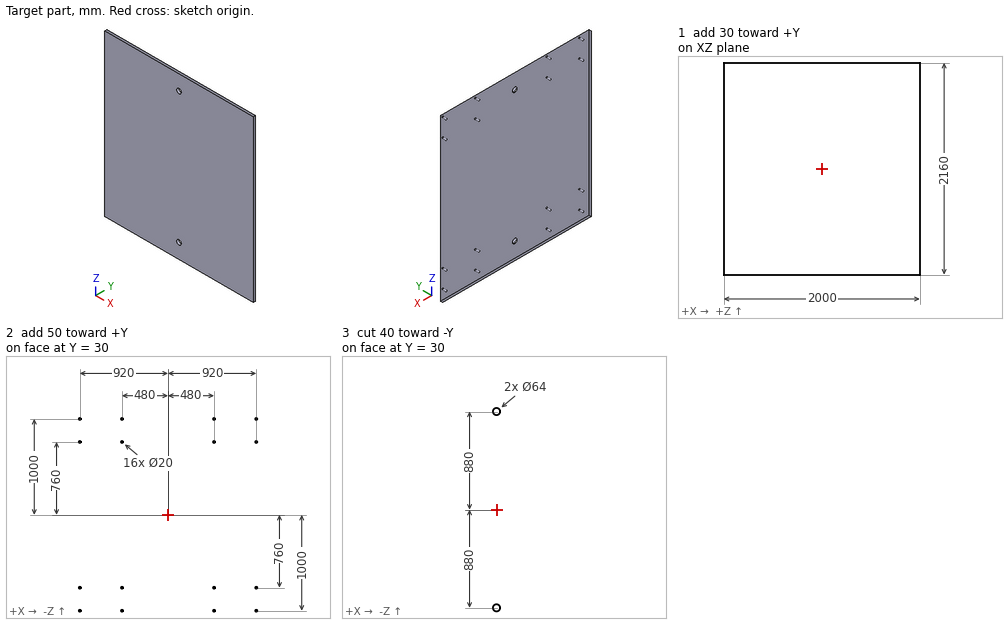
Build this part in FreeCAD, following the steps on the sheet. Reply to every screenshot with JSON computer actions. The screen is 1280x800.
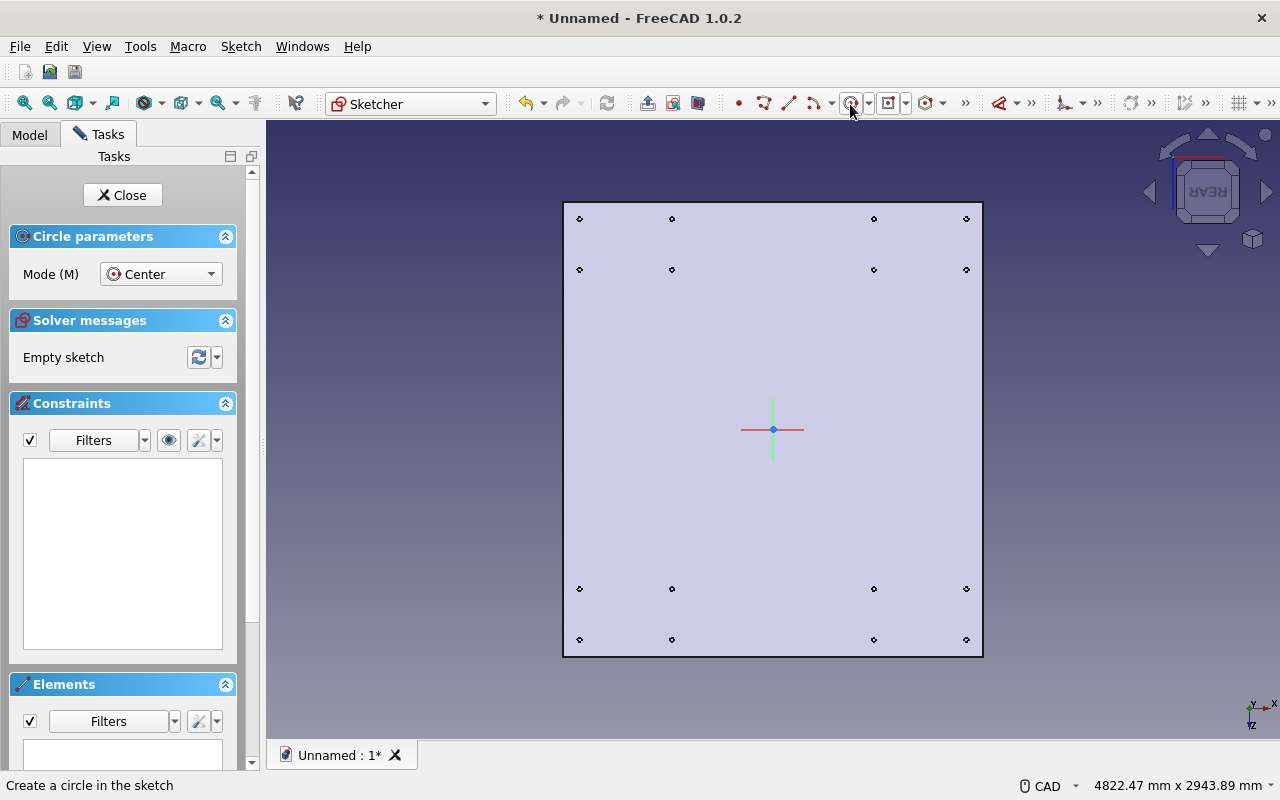
{"action": "scroll", "coordinate": [773, 244], "scroll_direction": "up", "scroll_amount": 7}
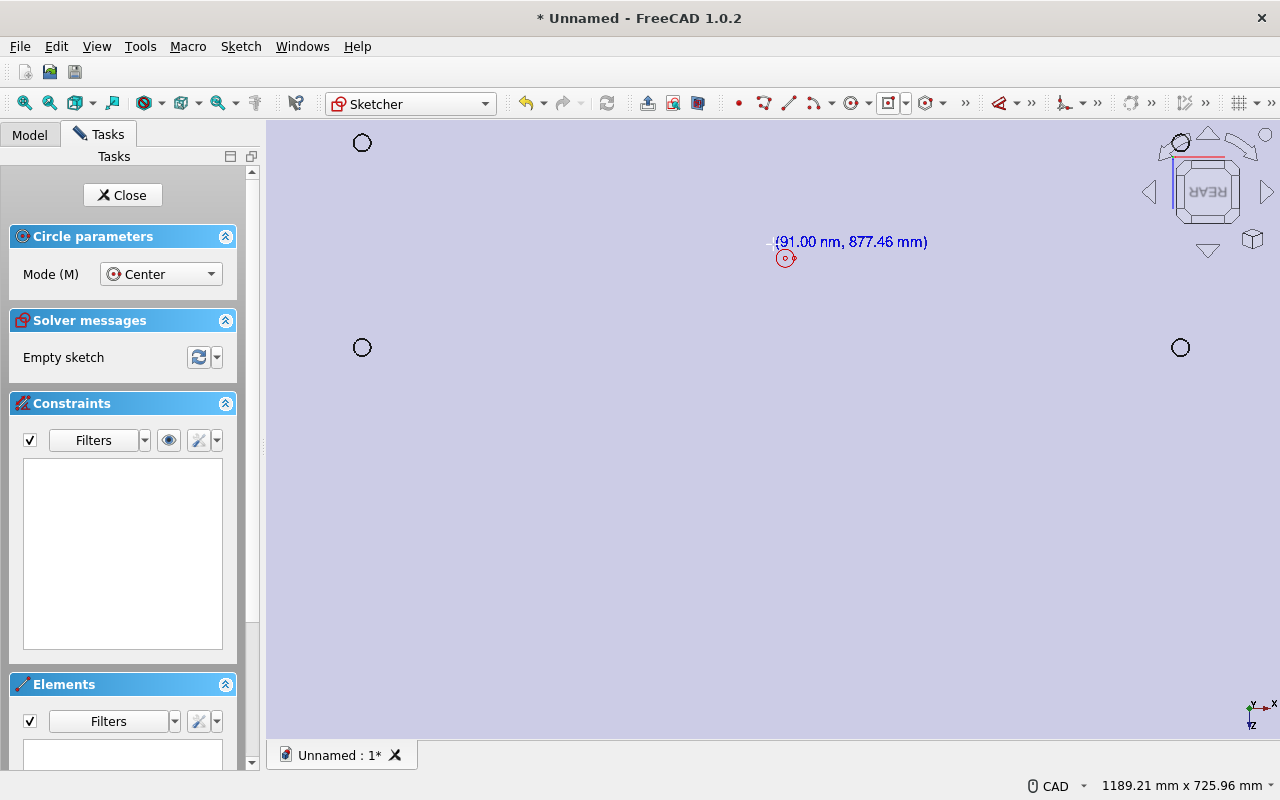
{"action": "scroll", "coordinate": [683, 244], "scroll_direction": "down", "scroll_amount": 7}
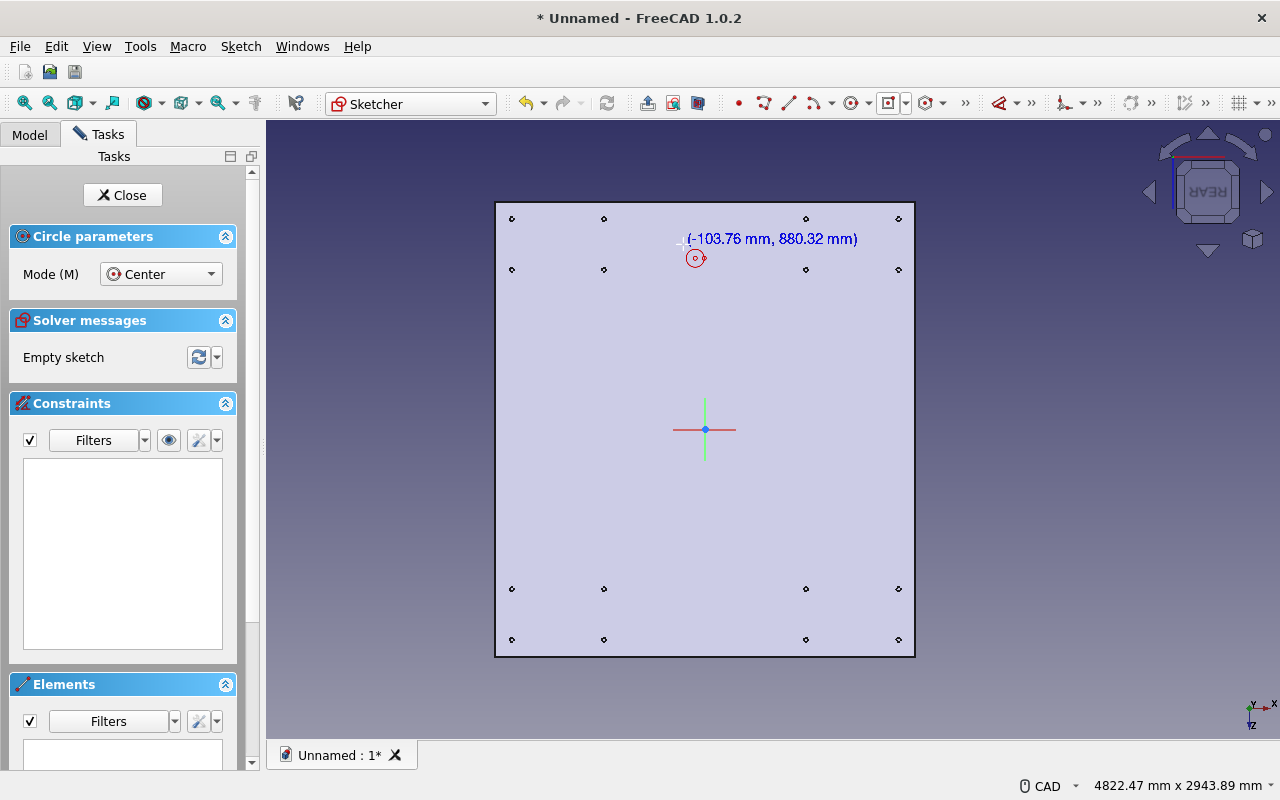
{"action": "left_click", "coordinate": [705, 244]}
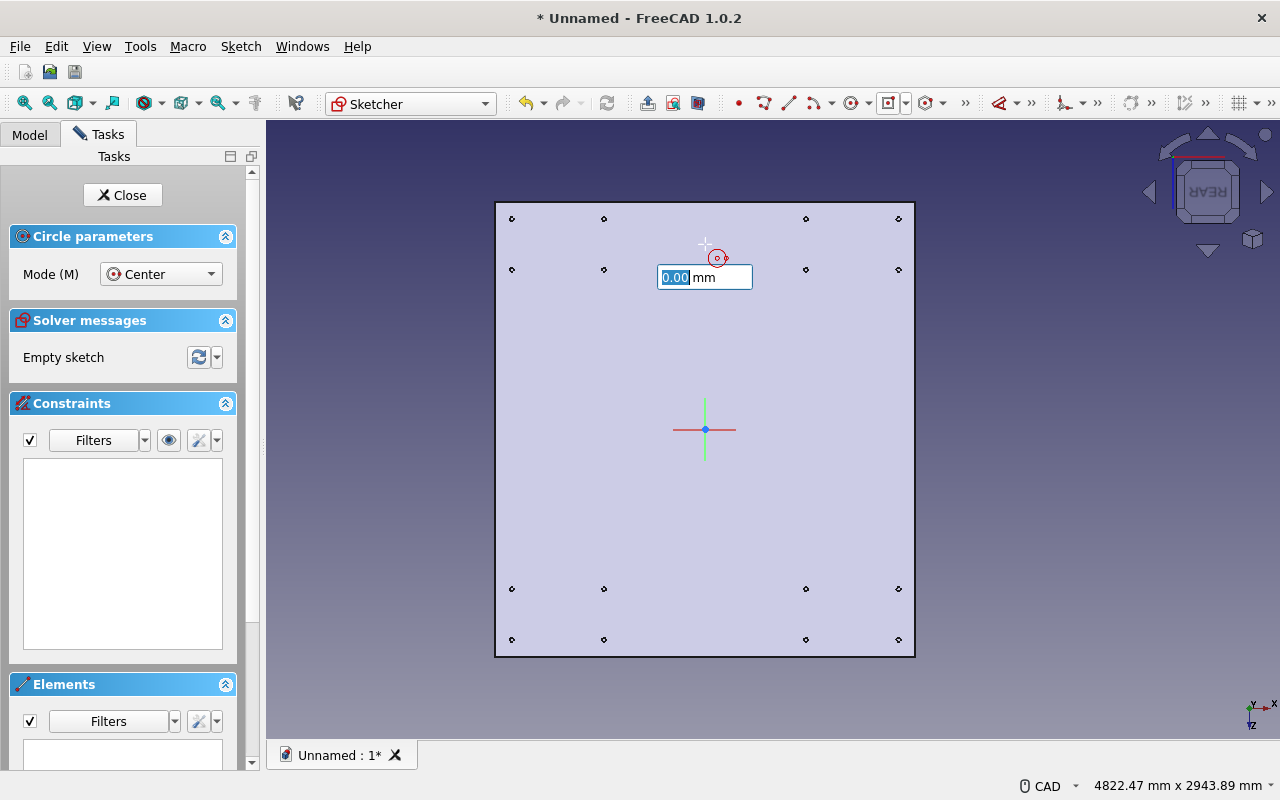
{"action": "scroll", "coordinate": [711, 242], "scroll_direction": "up", "scroll_amount": 5}
{"action": "mouse_move", "coordinate": [711, 242]}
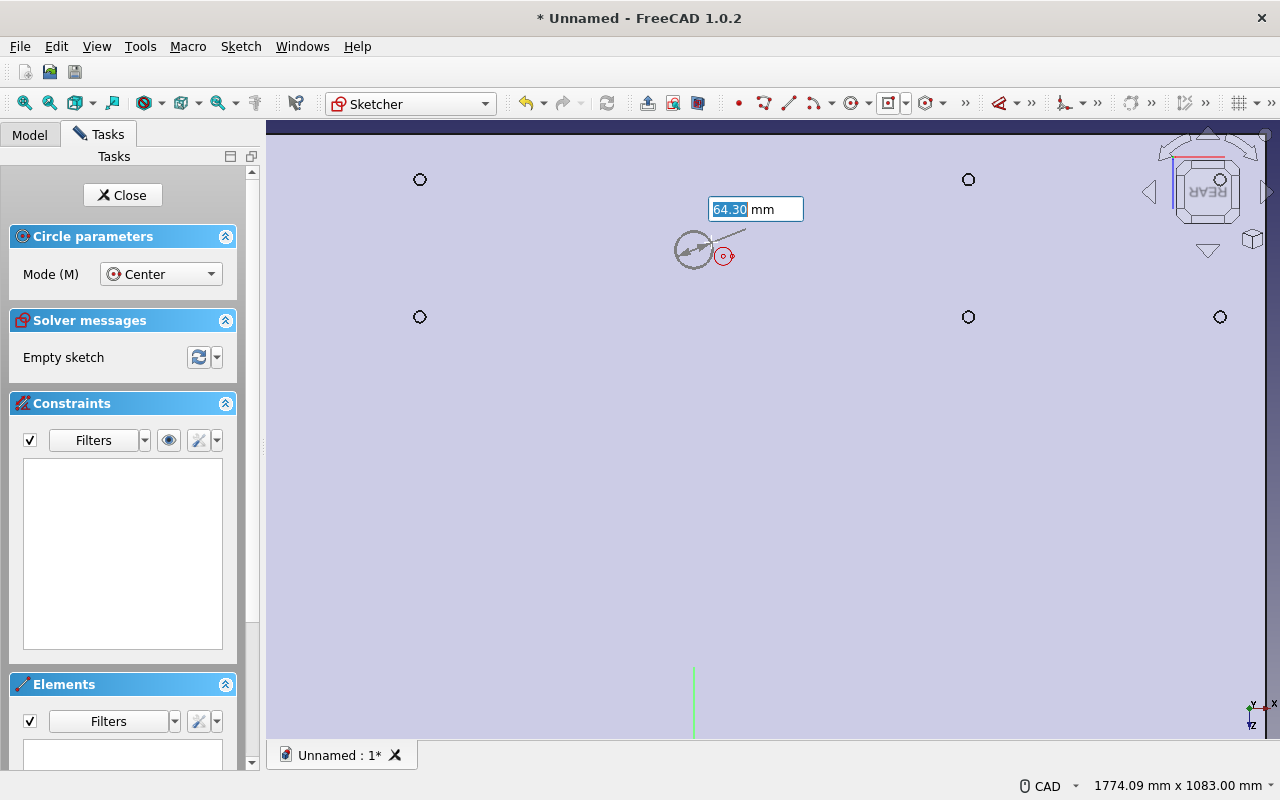
{"action": "type", "text": "64"}
{"action": "key", "text": "Return"}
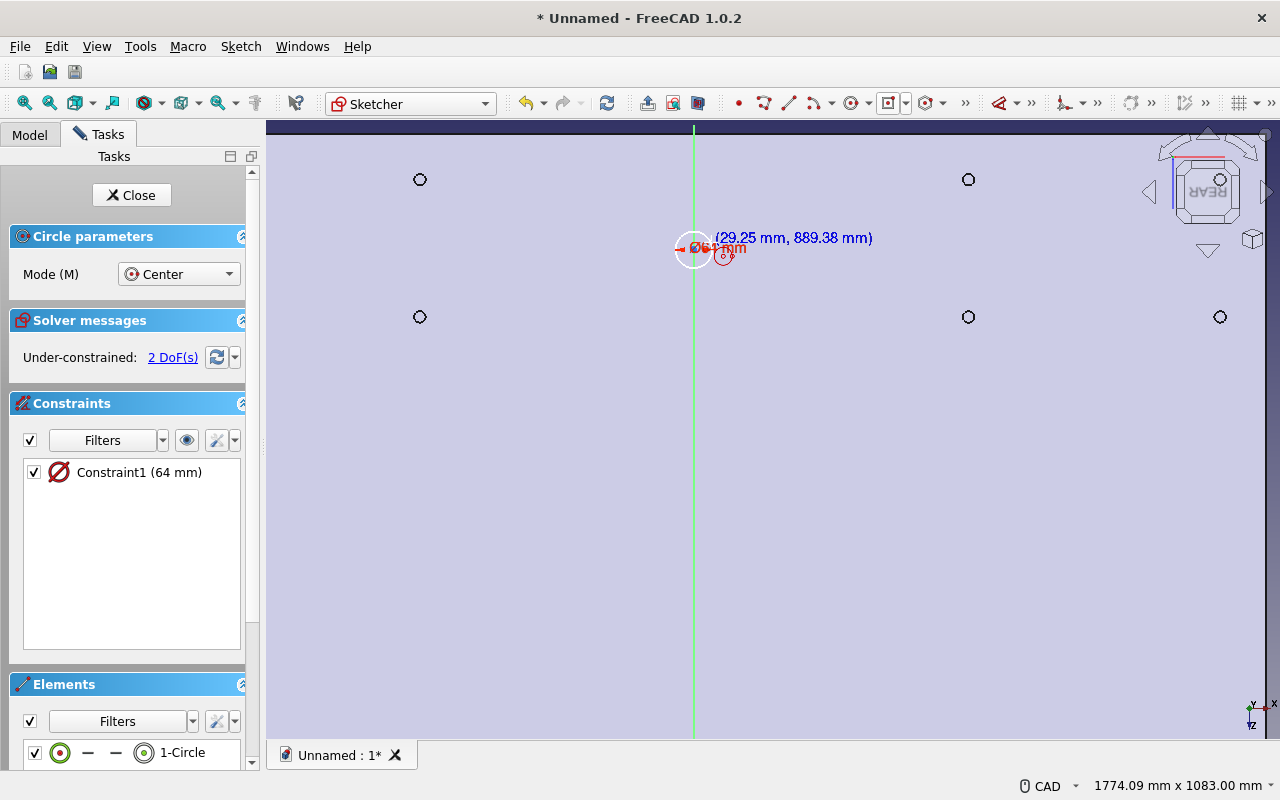
{"action": "scroll", "coordinate": [710, 242], "scroll_direction": "down", "scroll_amount": 5}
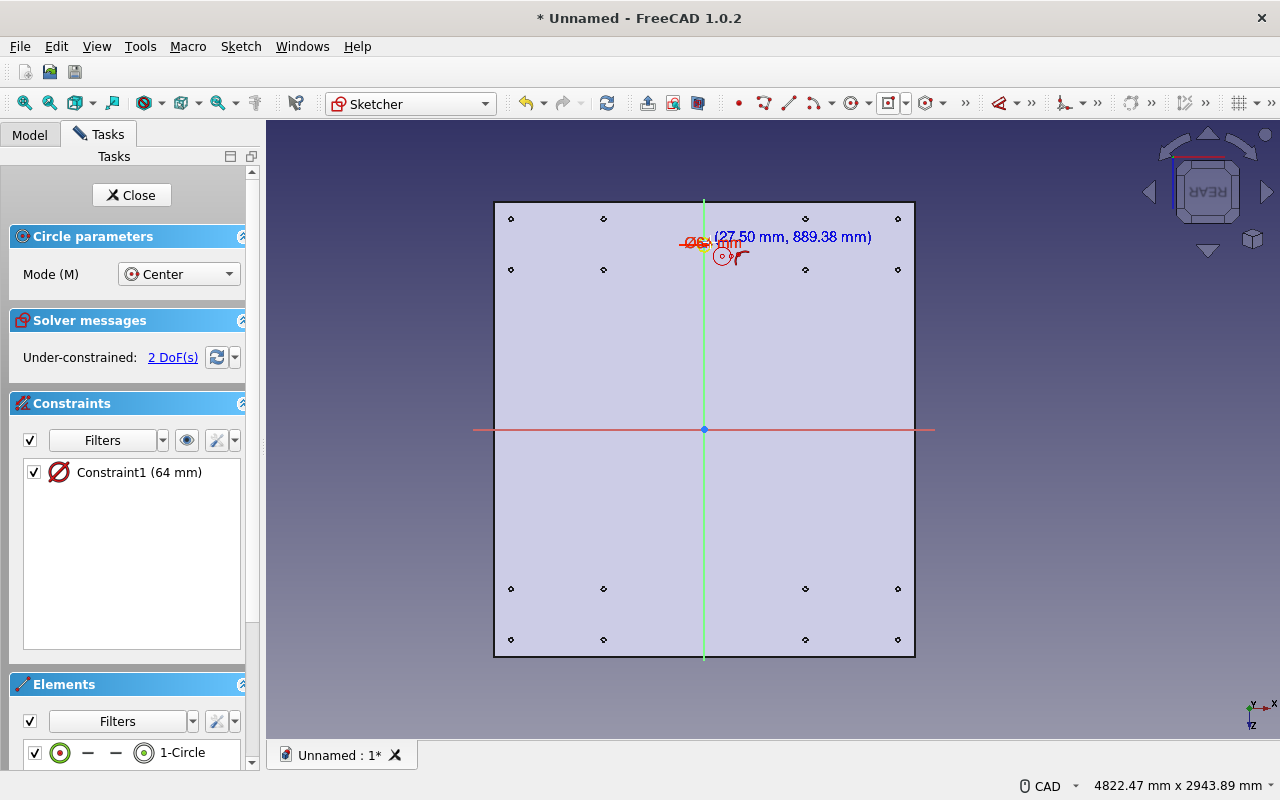
{"action": "scroll", "coordinate": [704, 615], "scroll_direction": "up", "scroll_amount": 7}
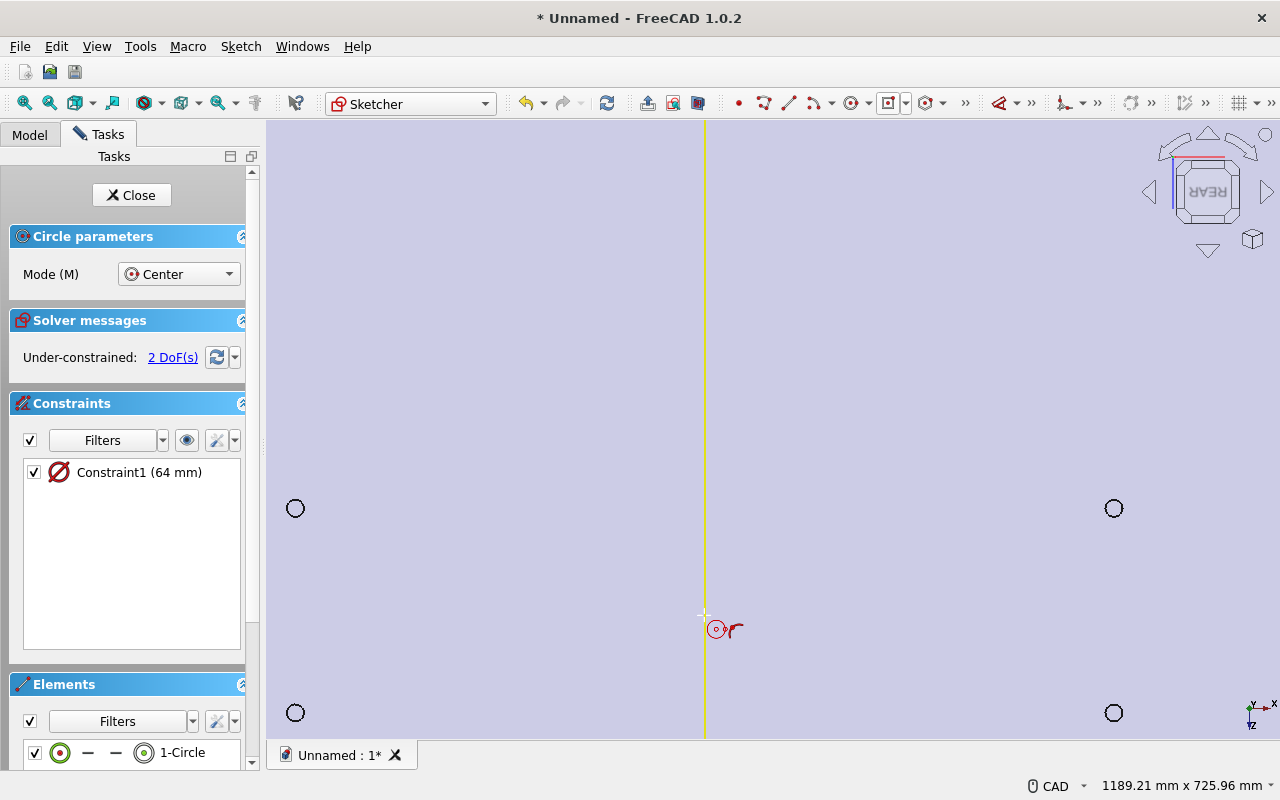
{"action": "scroll", "coordinate": [704, 616], "scroll_direction": "down", "scroll_amount": 7}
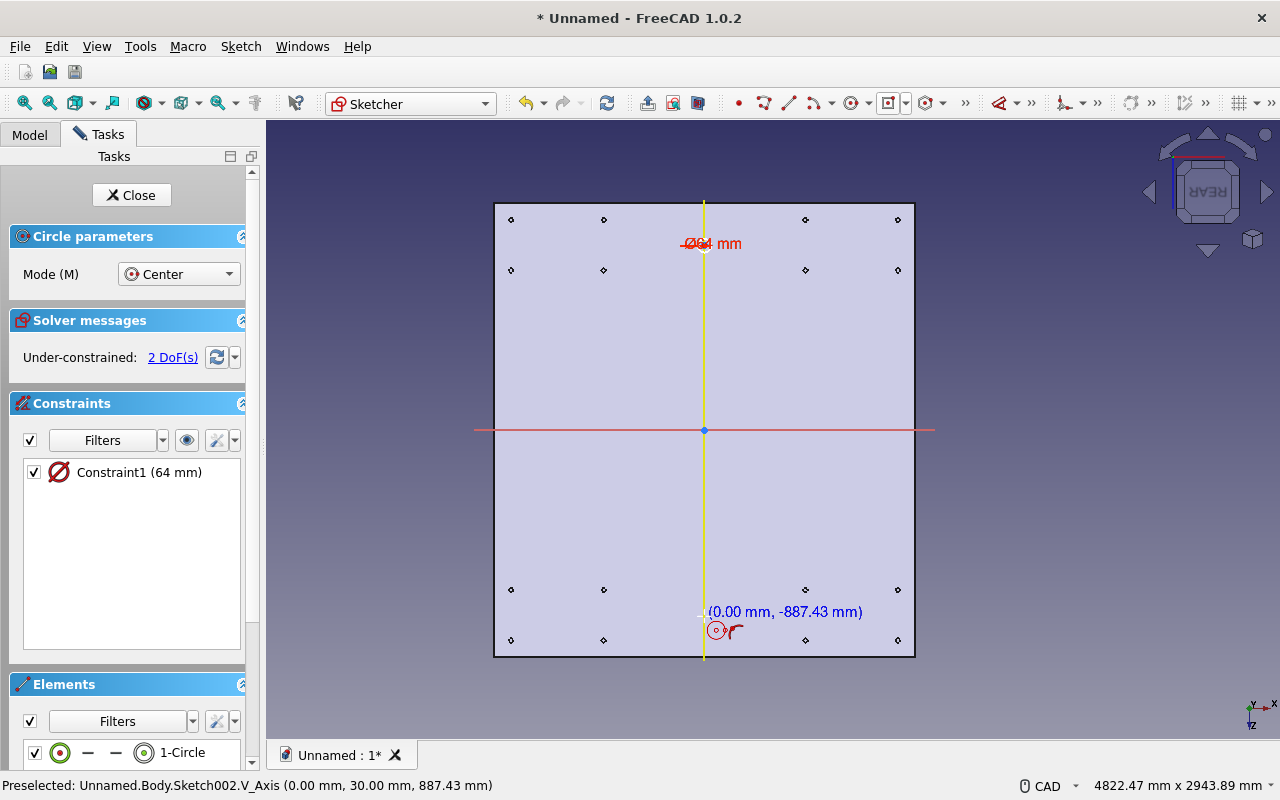
{"action": "left_click", "coordinate": [704, 615]}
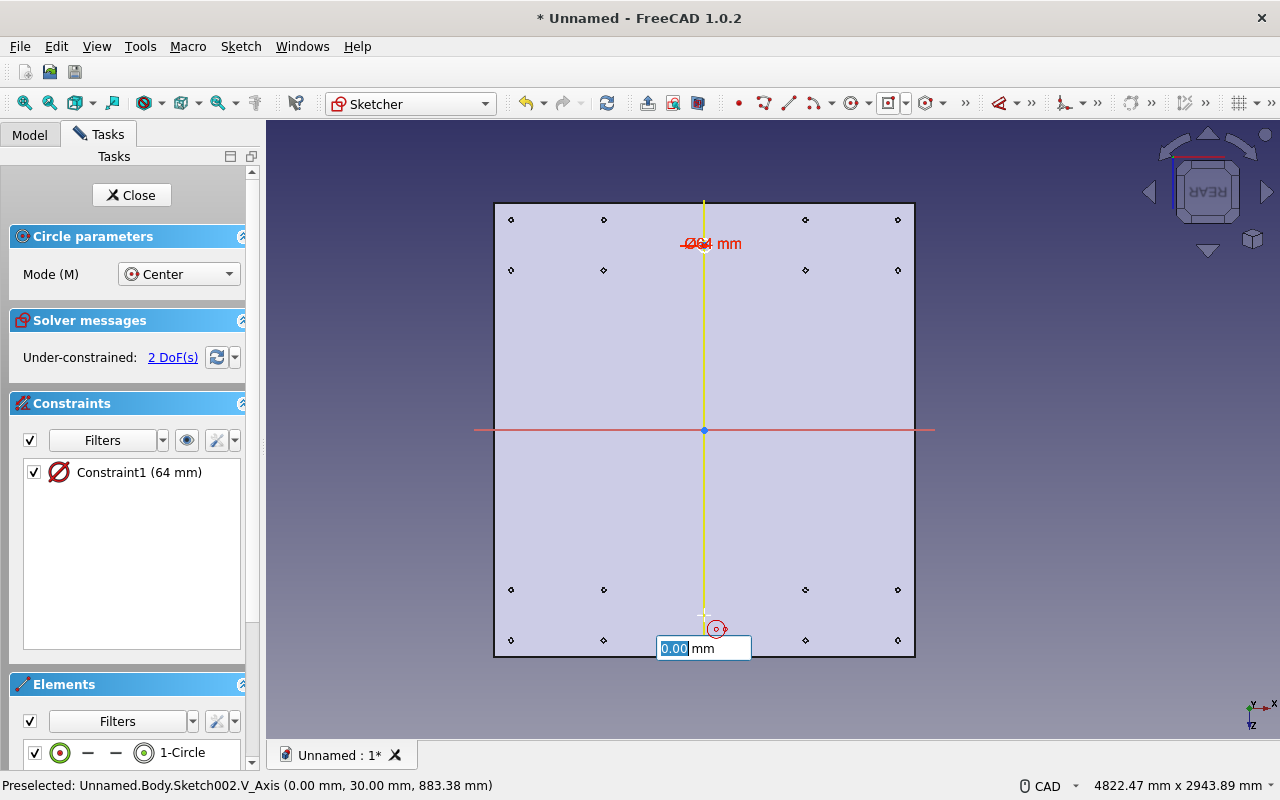
{"action": "scroll", "coordinate": [711, 613], "scroll_direction": "up", "scroll_amount": 5}
{"action": "mouse_move", "coordinate": [710, 612]}